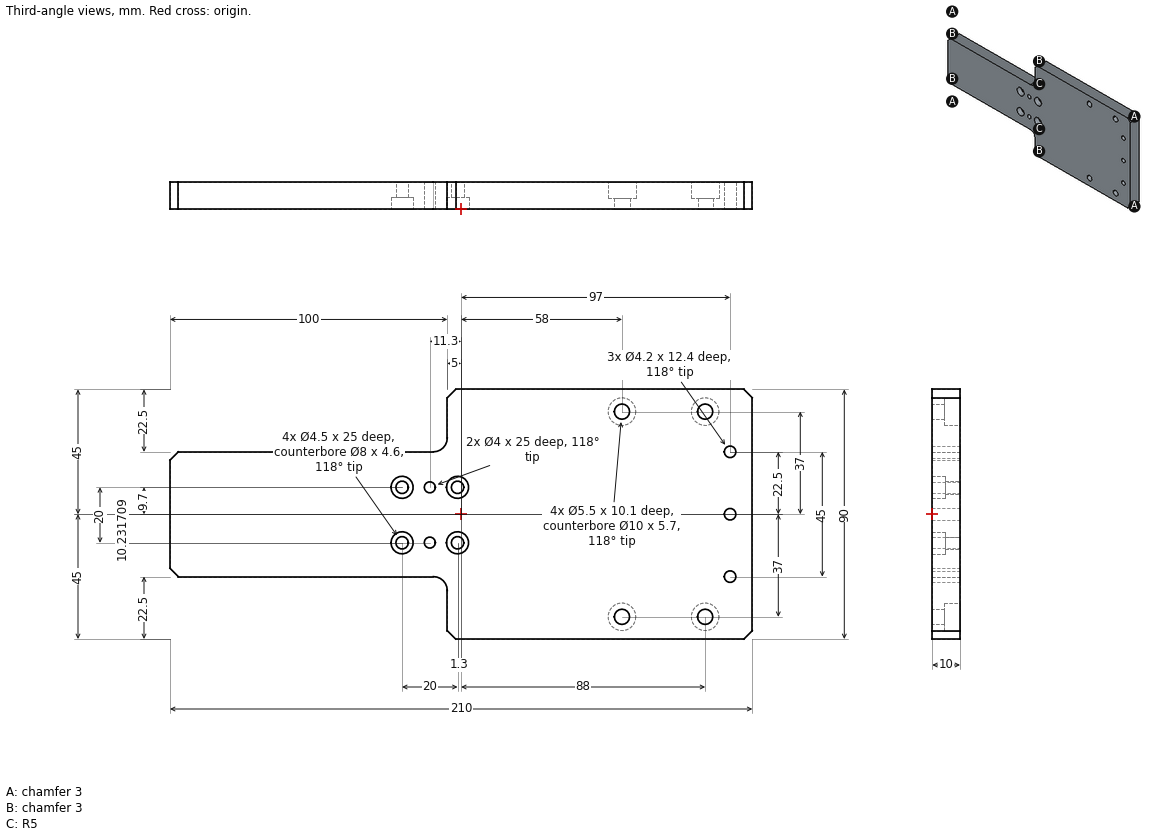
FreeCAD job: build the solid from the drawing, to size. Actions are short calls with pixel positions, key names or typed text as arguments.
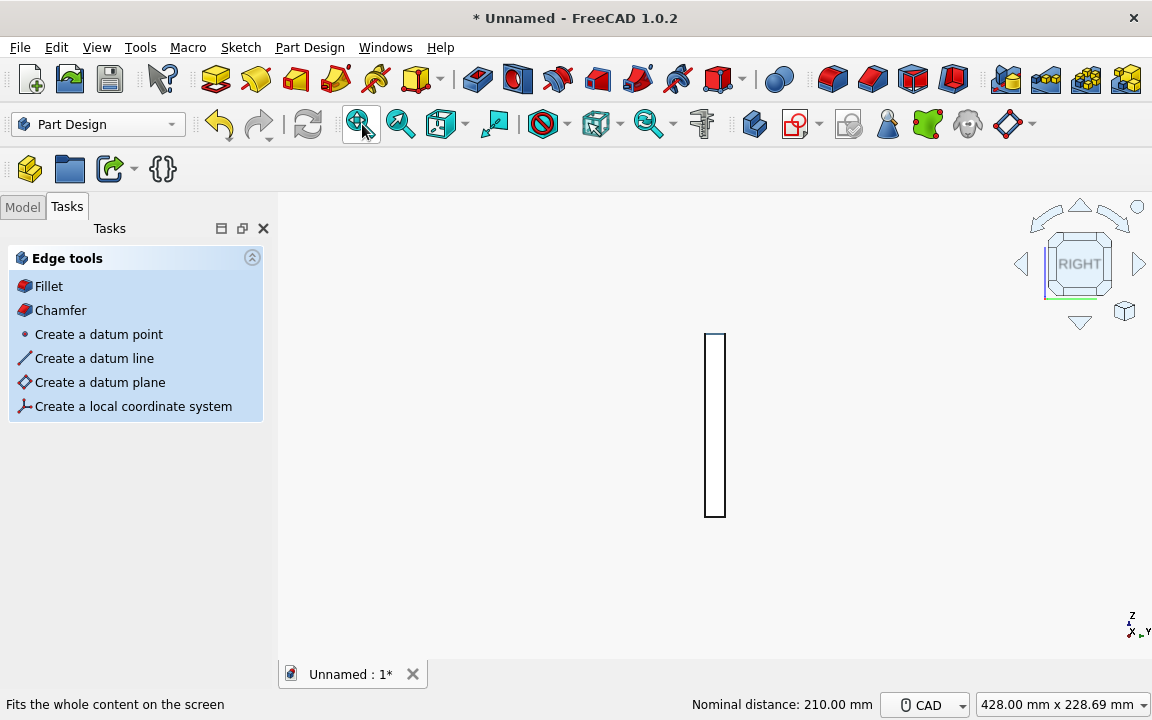
click(362, 124)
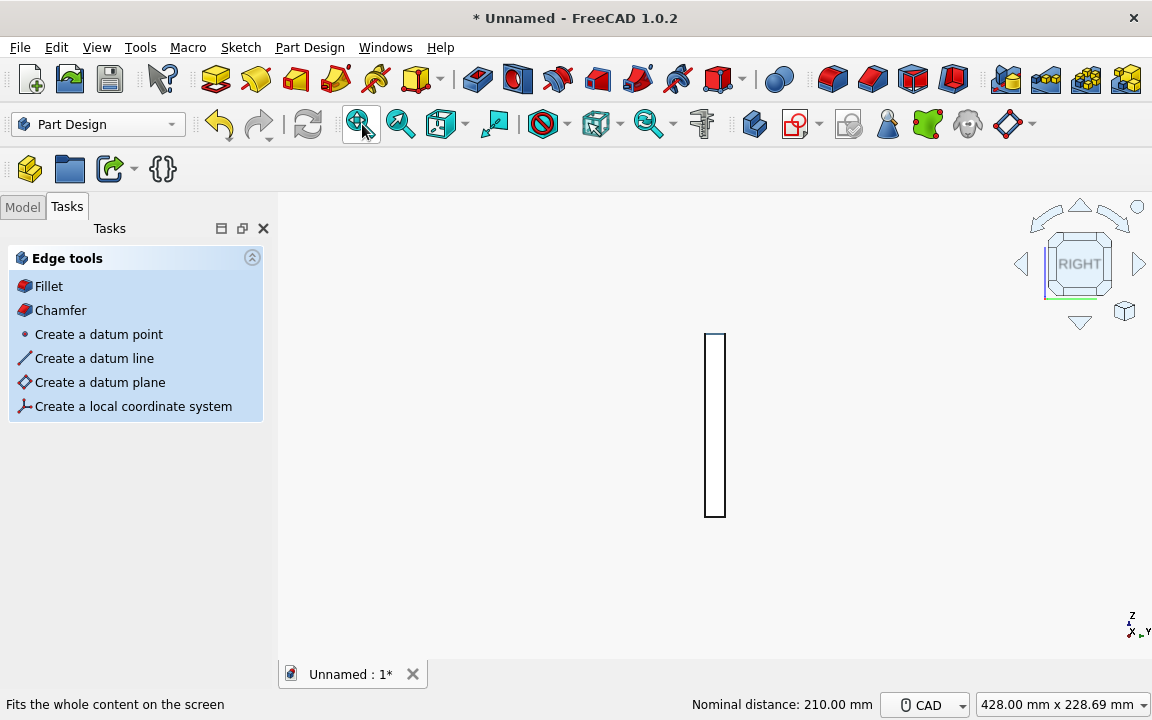
click(715, 516, ctrl)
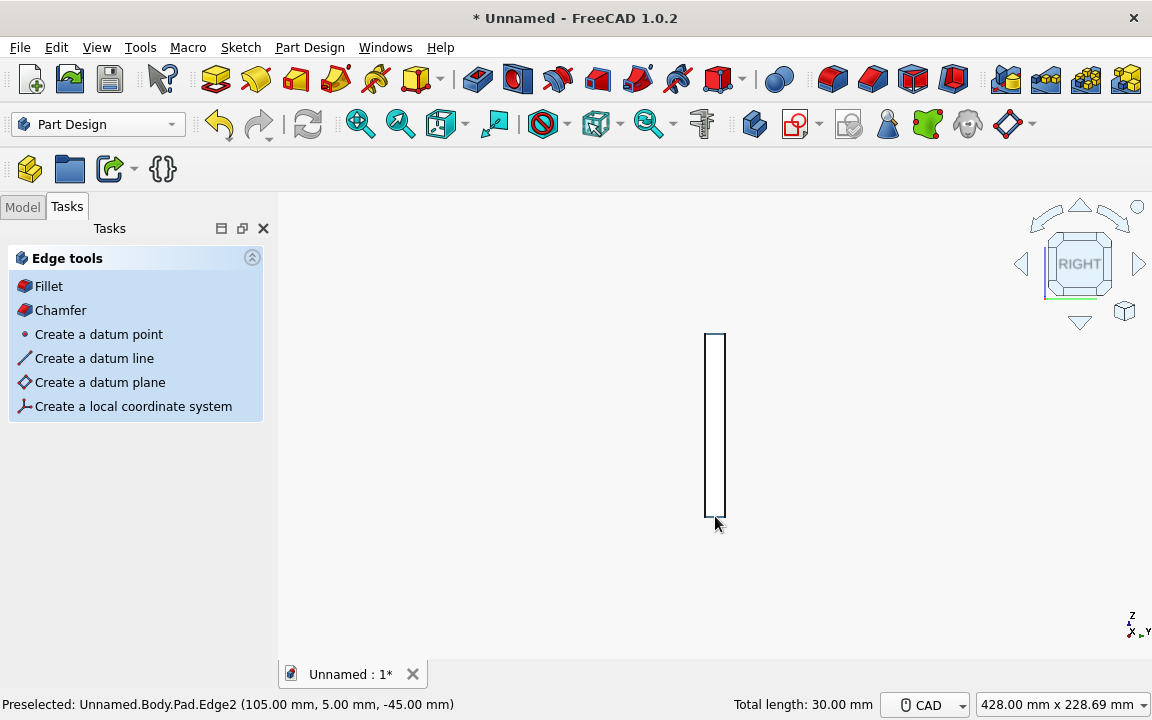
scroll(715, 516, up, 4)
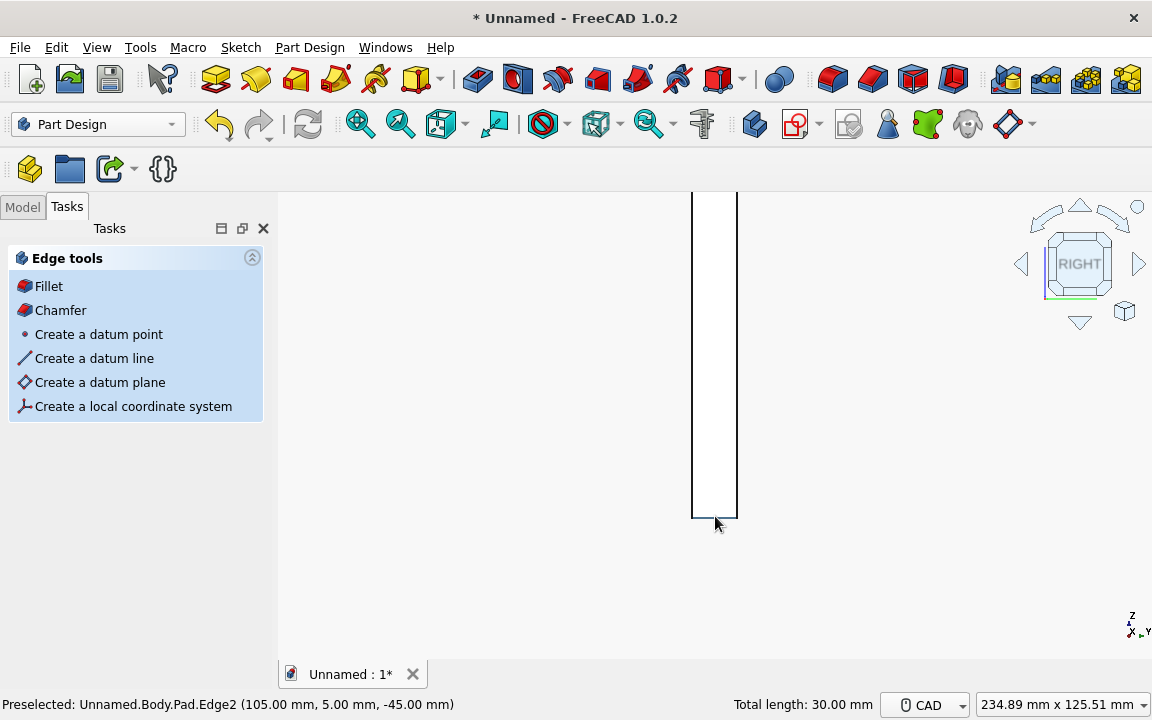
click(362, 124)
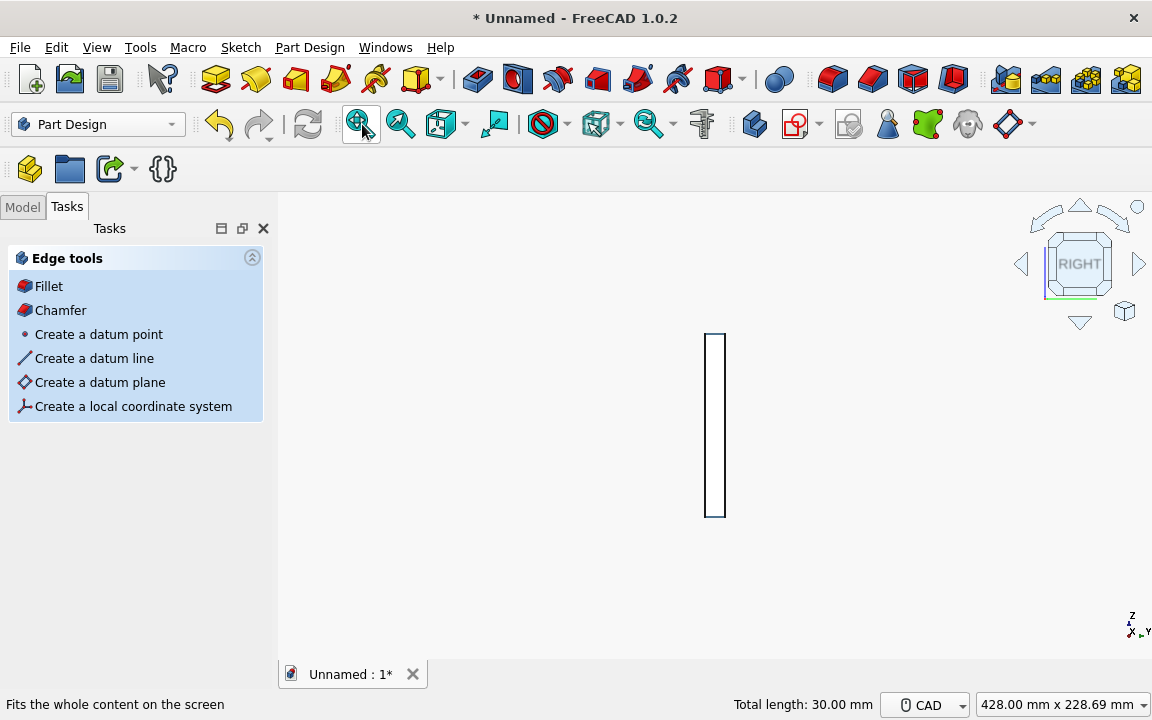
key(5)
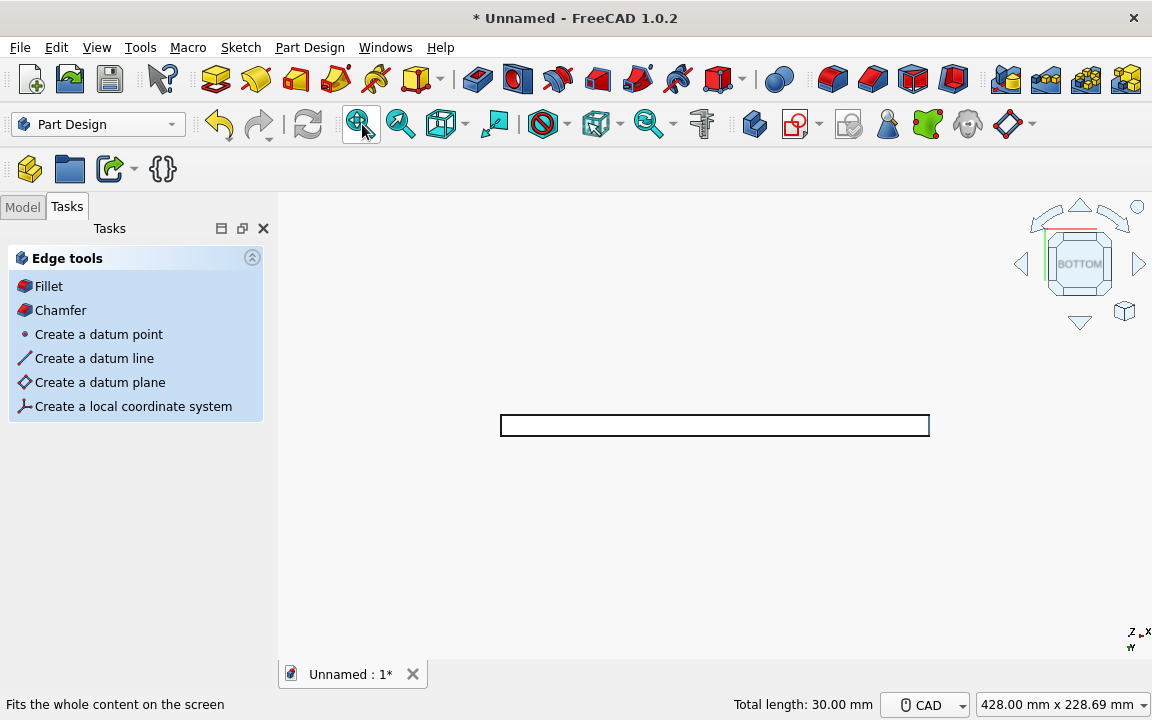
click(501, 424, ctrl)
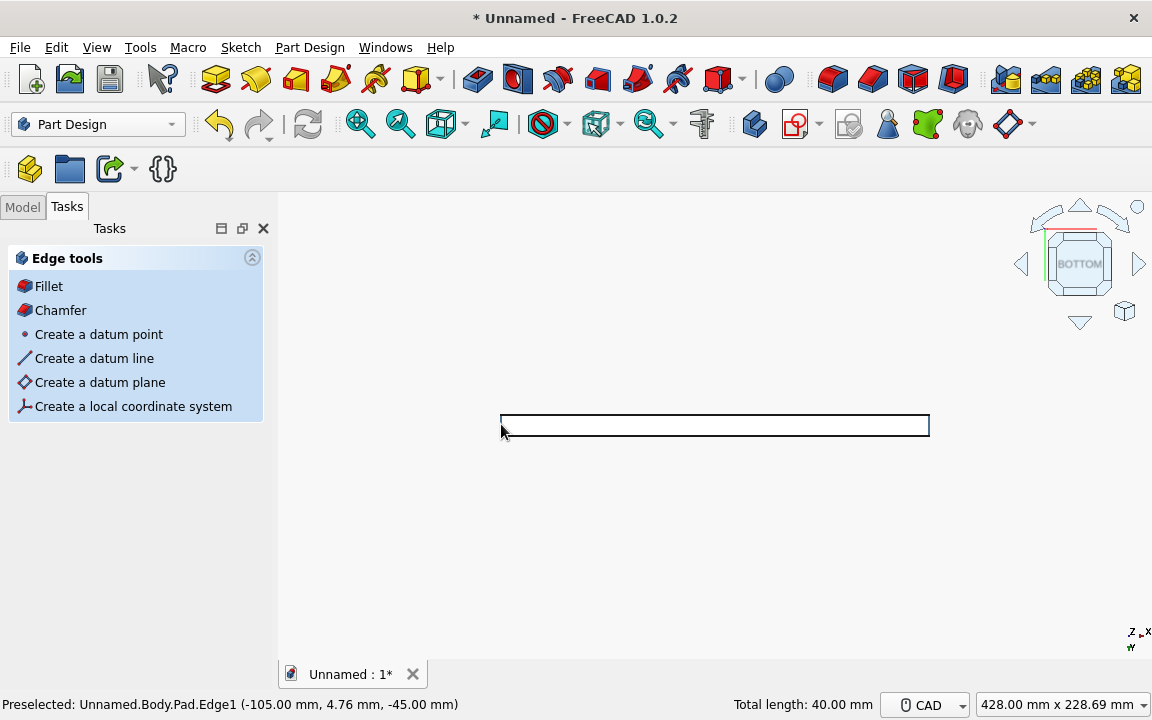
click(874, 80)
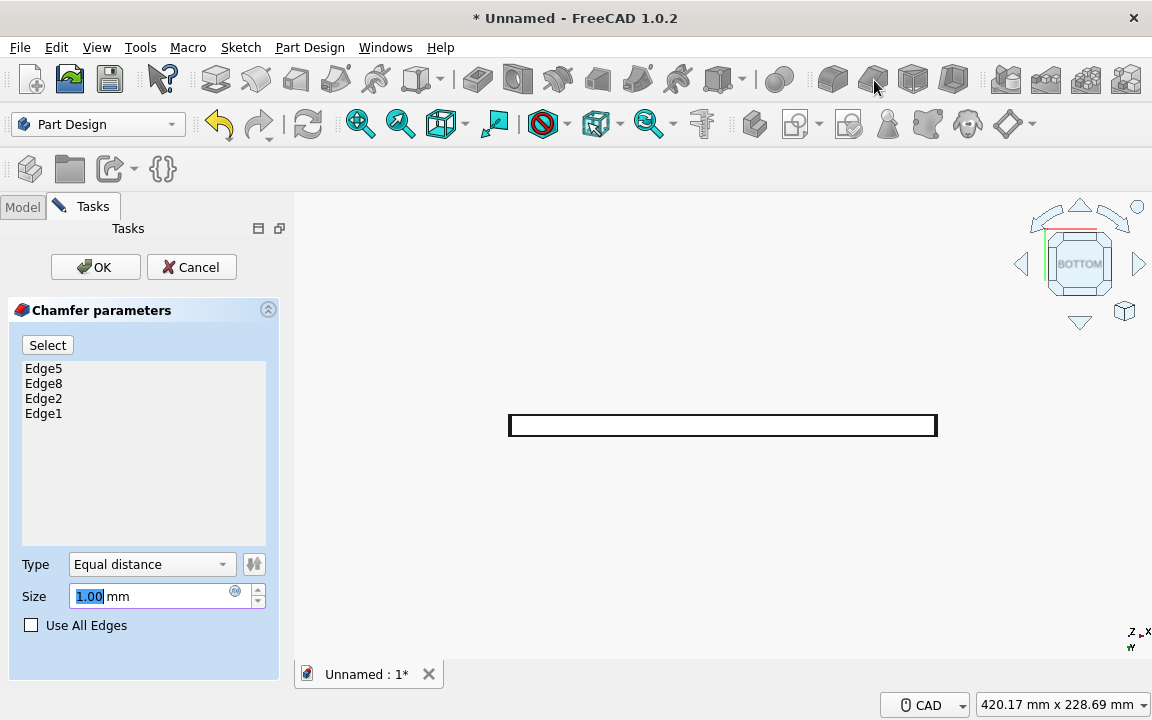
text(3)
key(Tab)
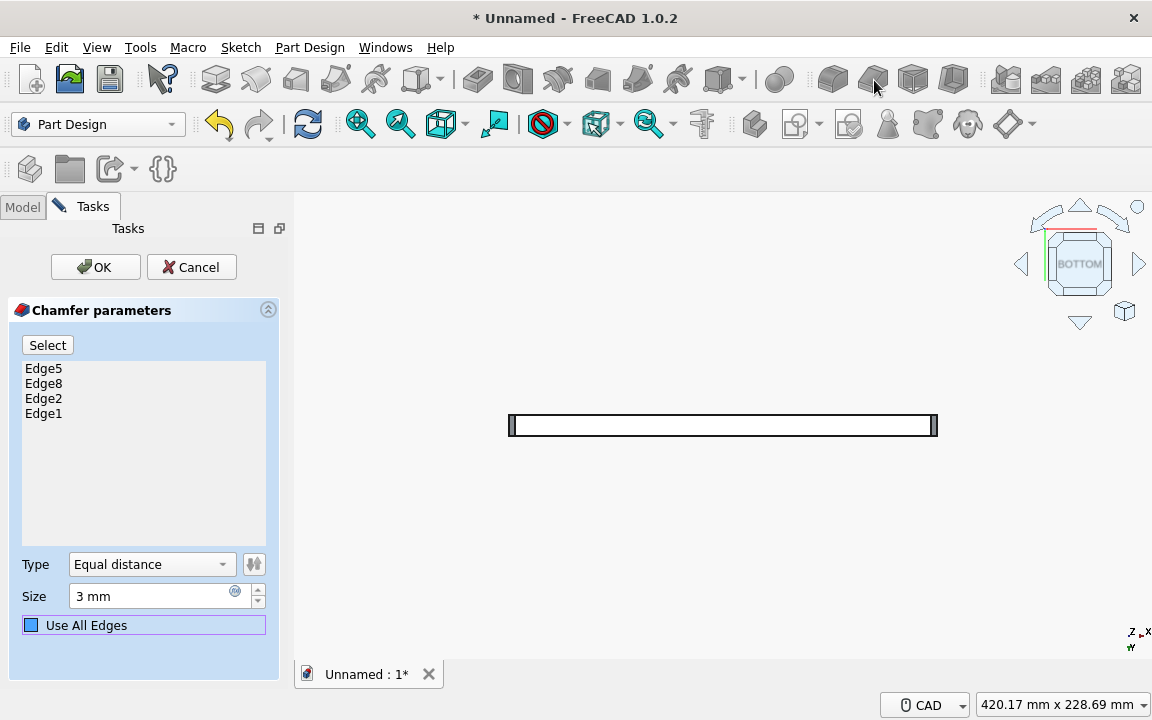
click(96, 267)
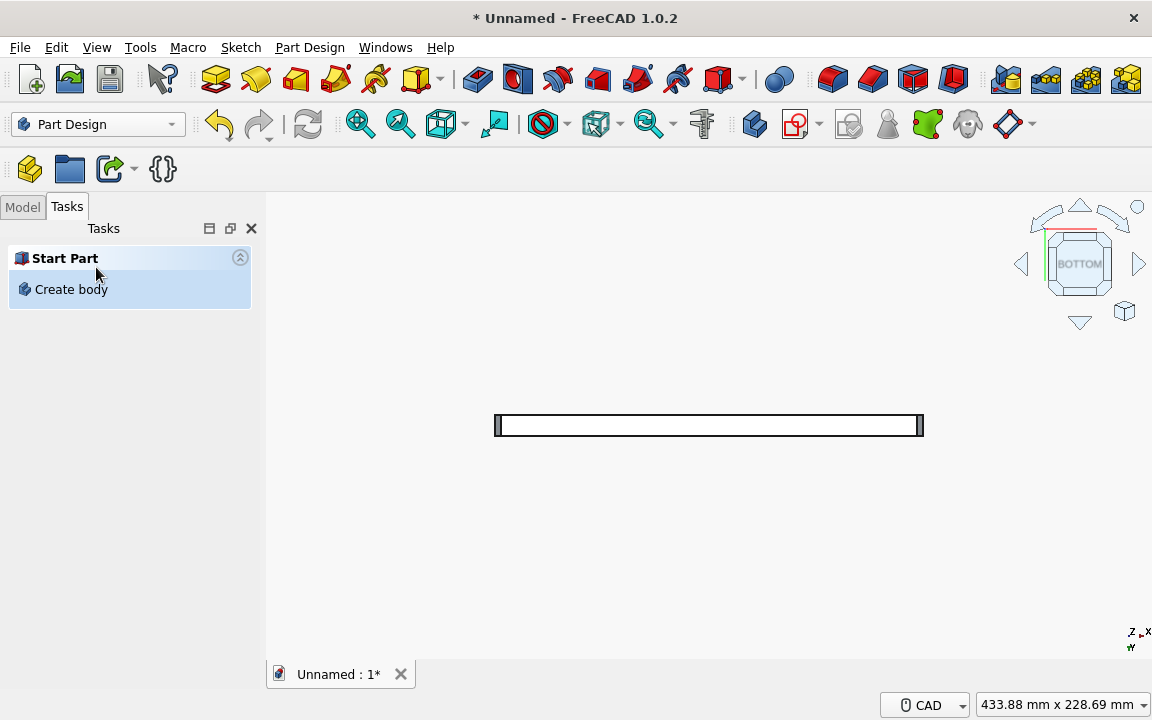
key(4)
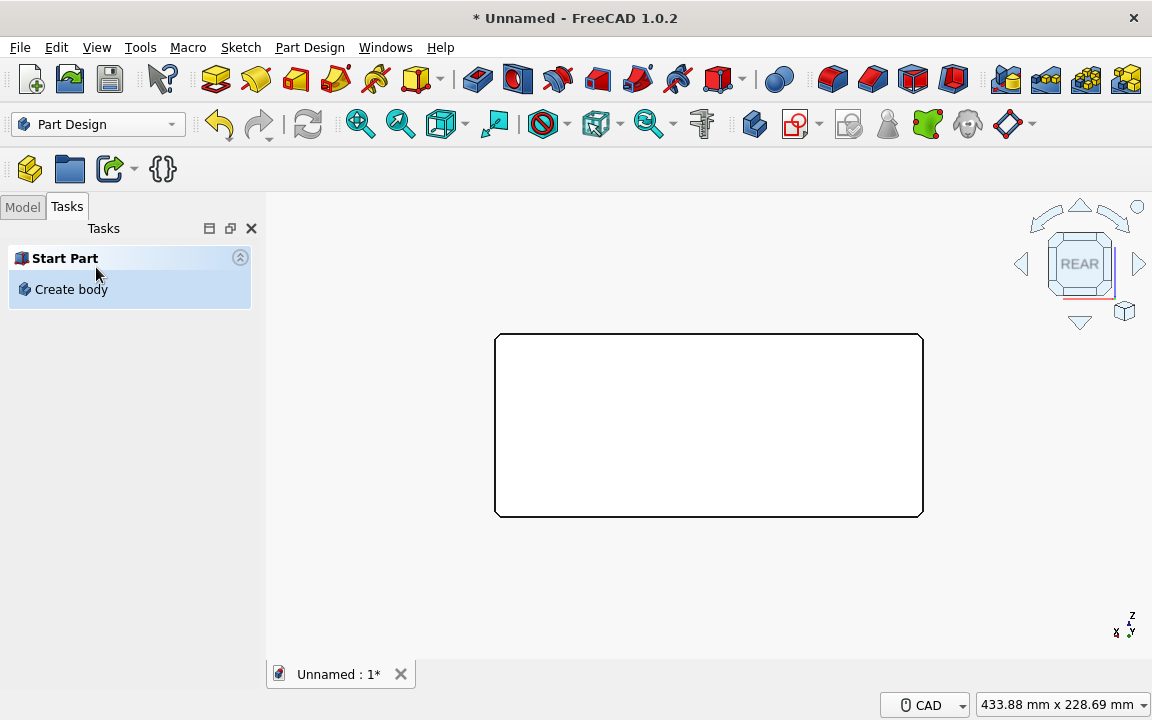
click(586, 424)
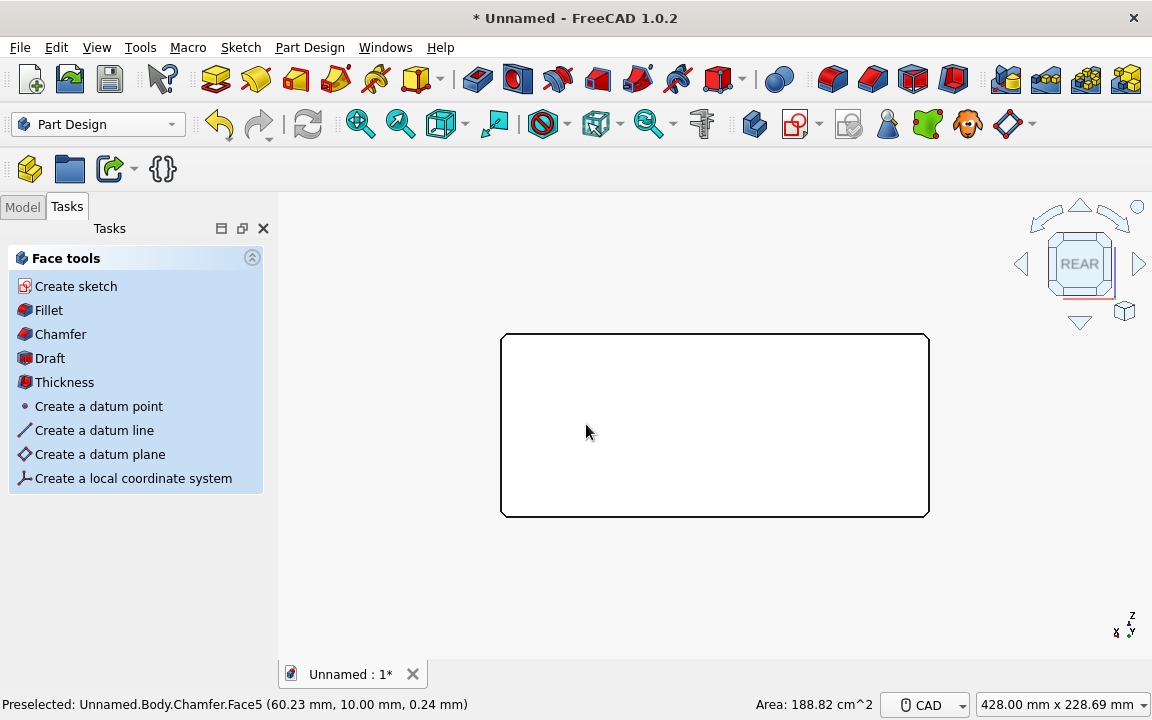
click(796, 124)